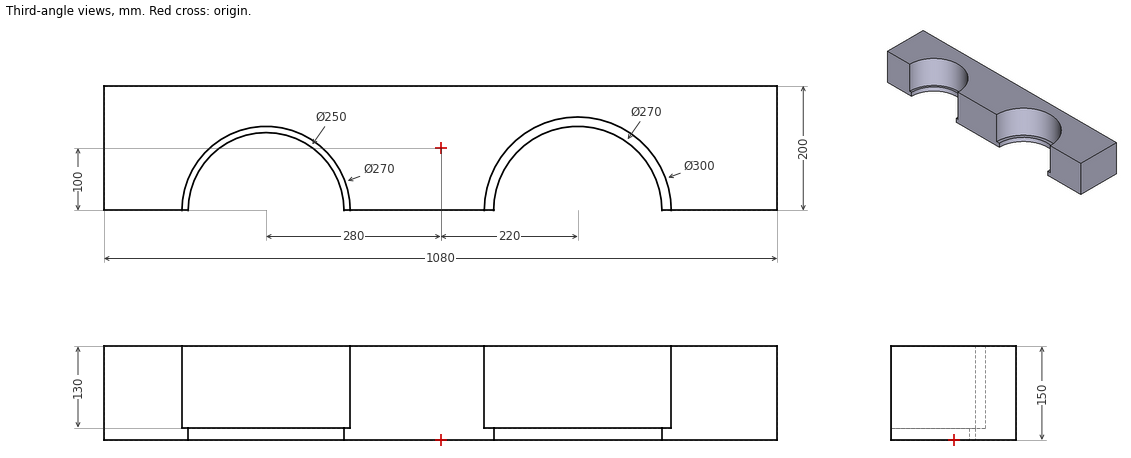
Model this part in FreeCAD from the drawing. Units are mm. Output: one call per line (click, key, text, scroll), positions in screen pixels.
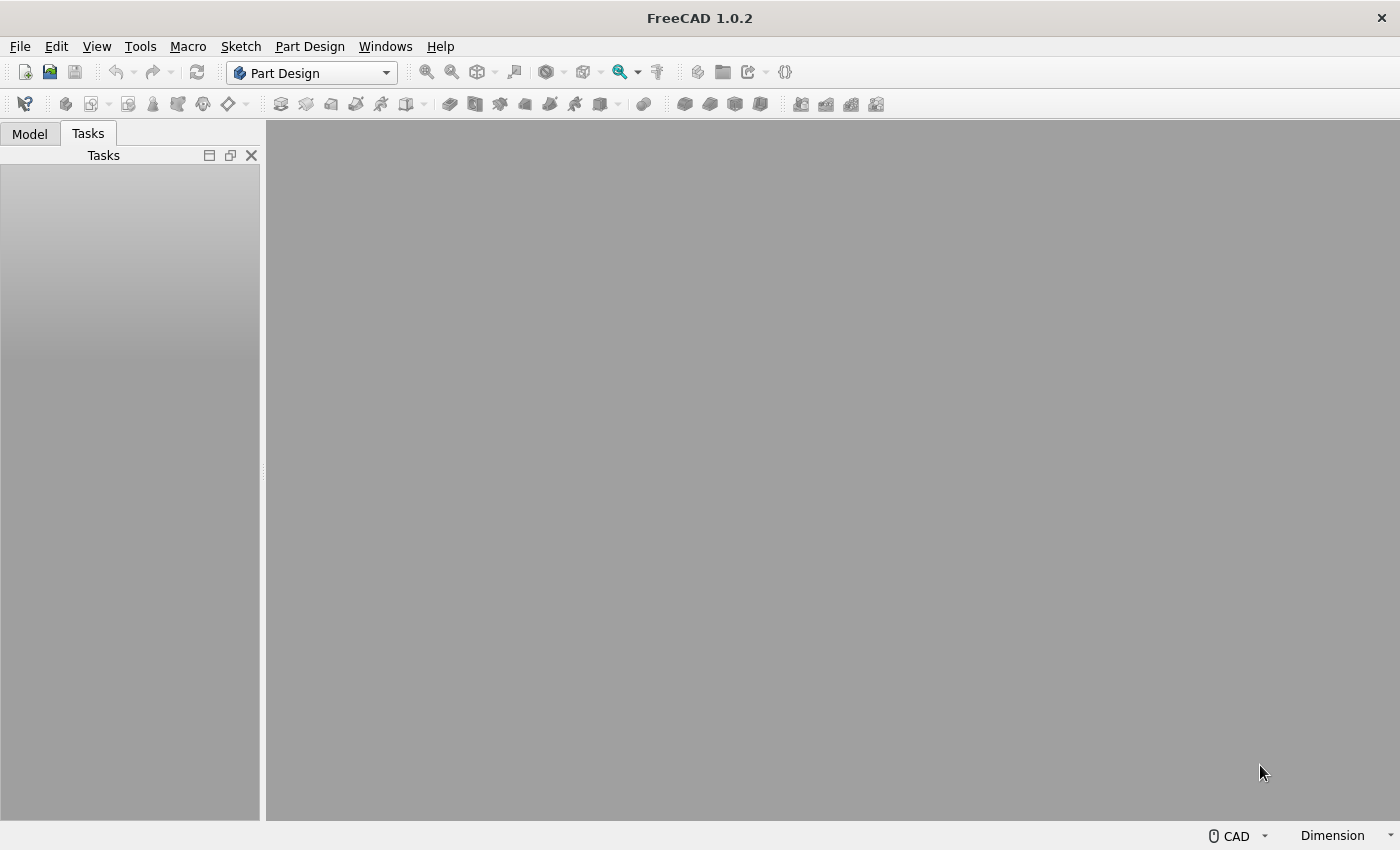
key(ctrl+n)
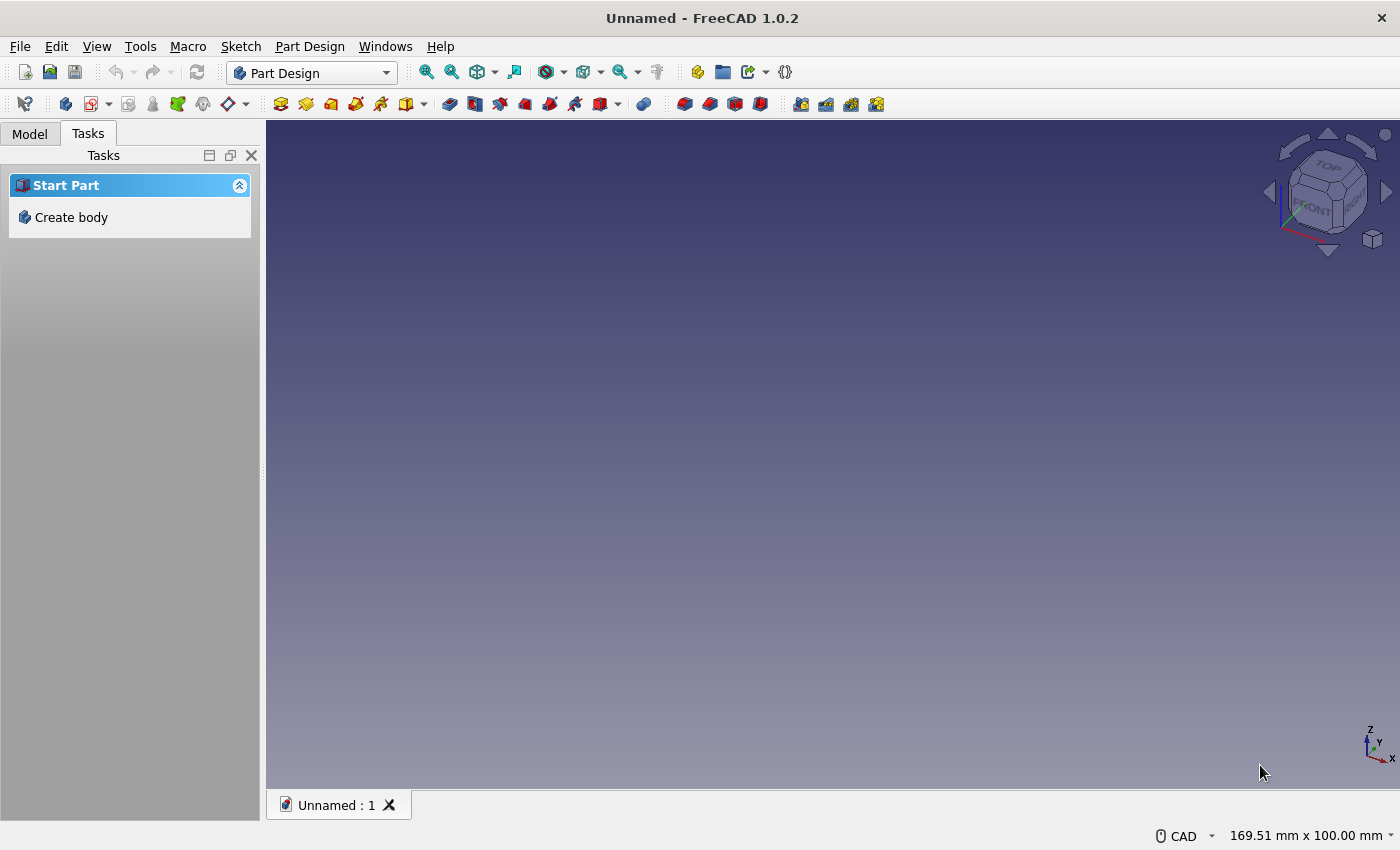
click(90, 104)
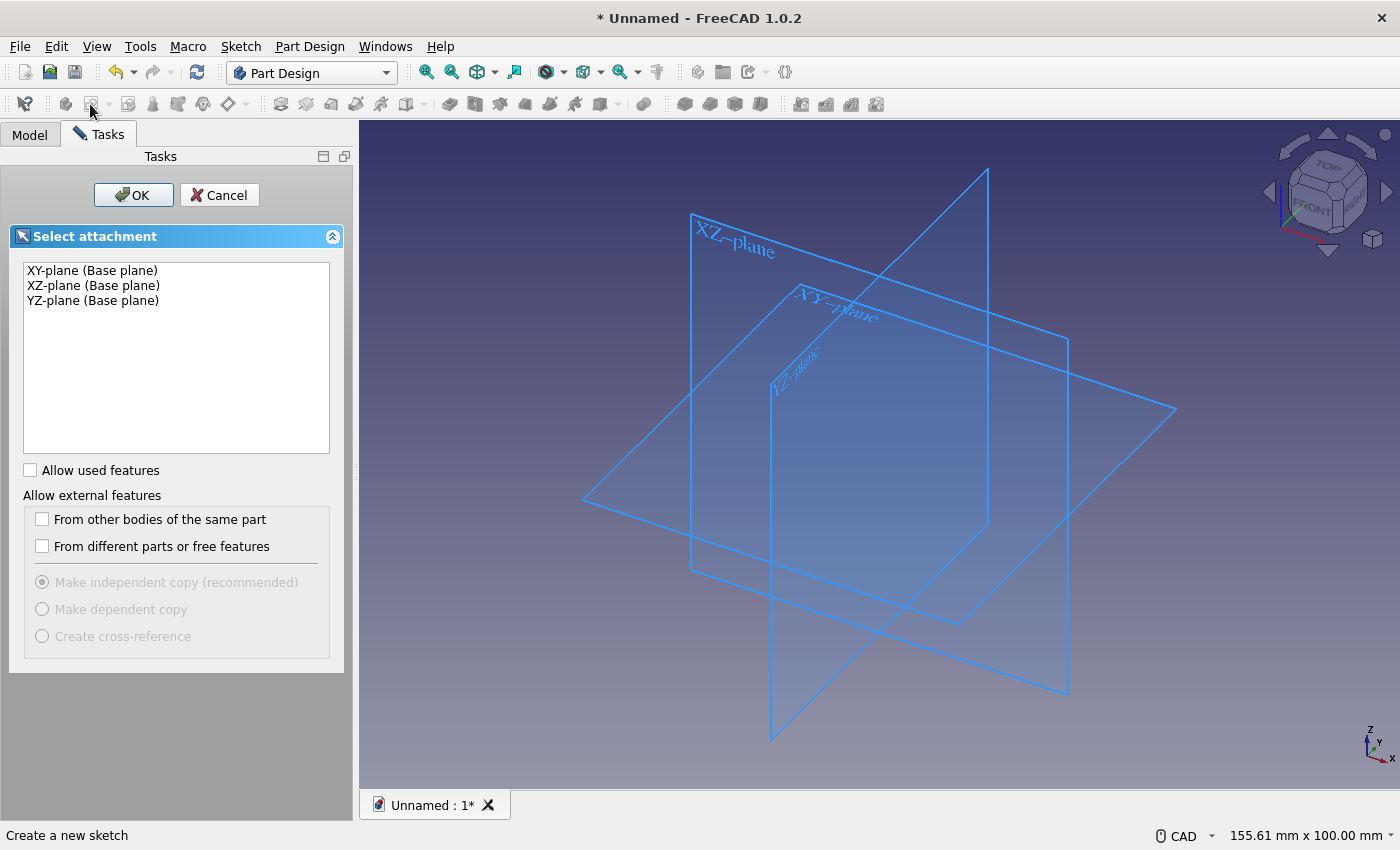
click(84, 270)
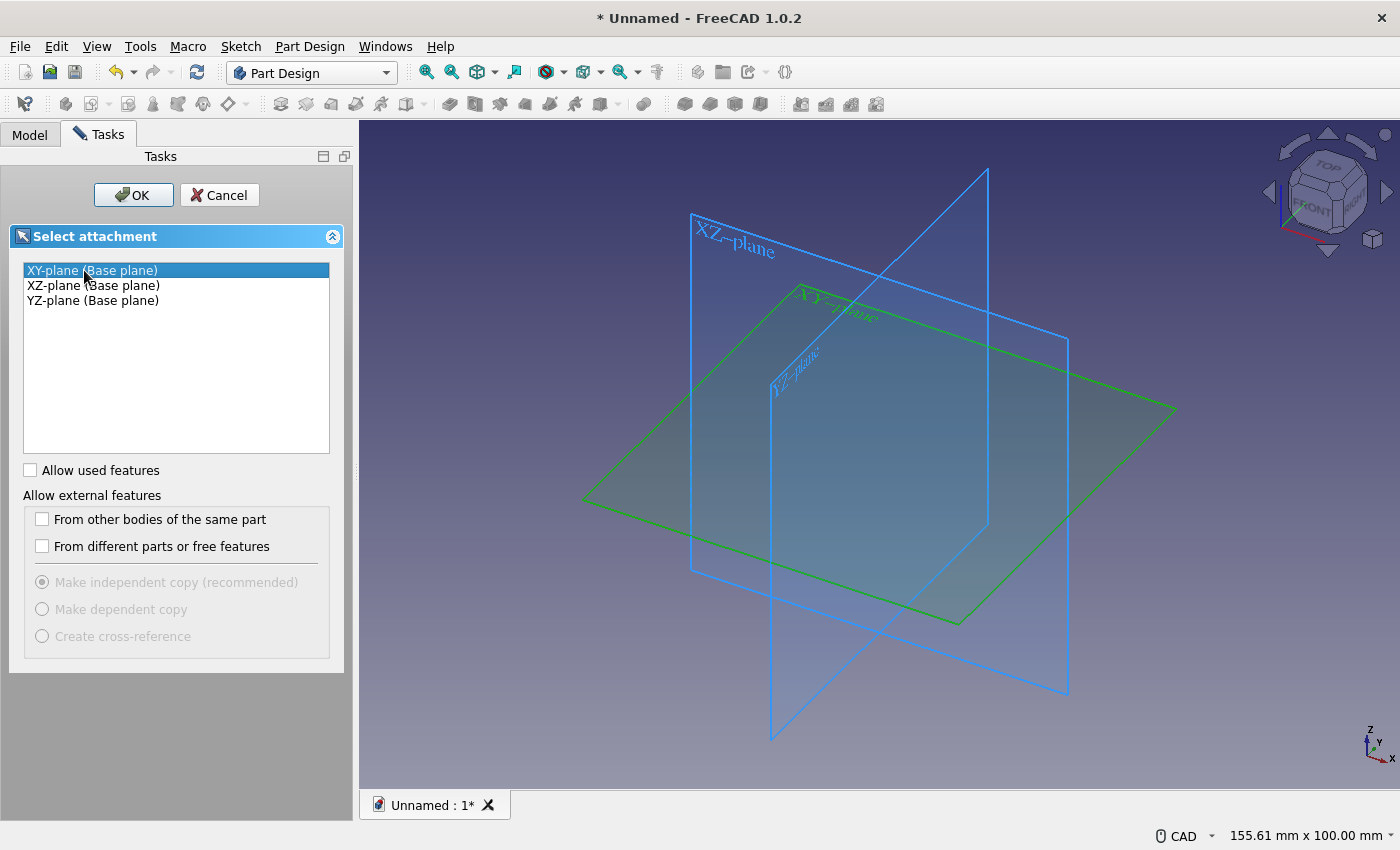
click(134, 195)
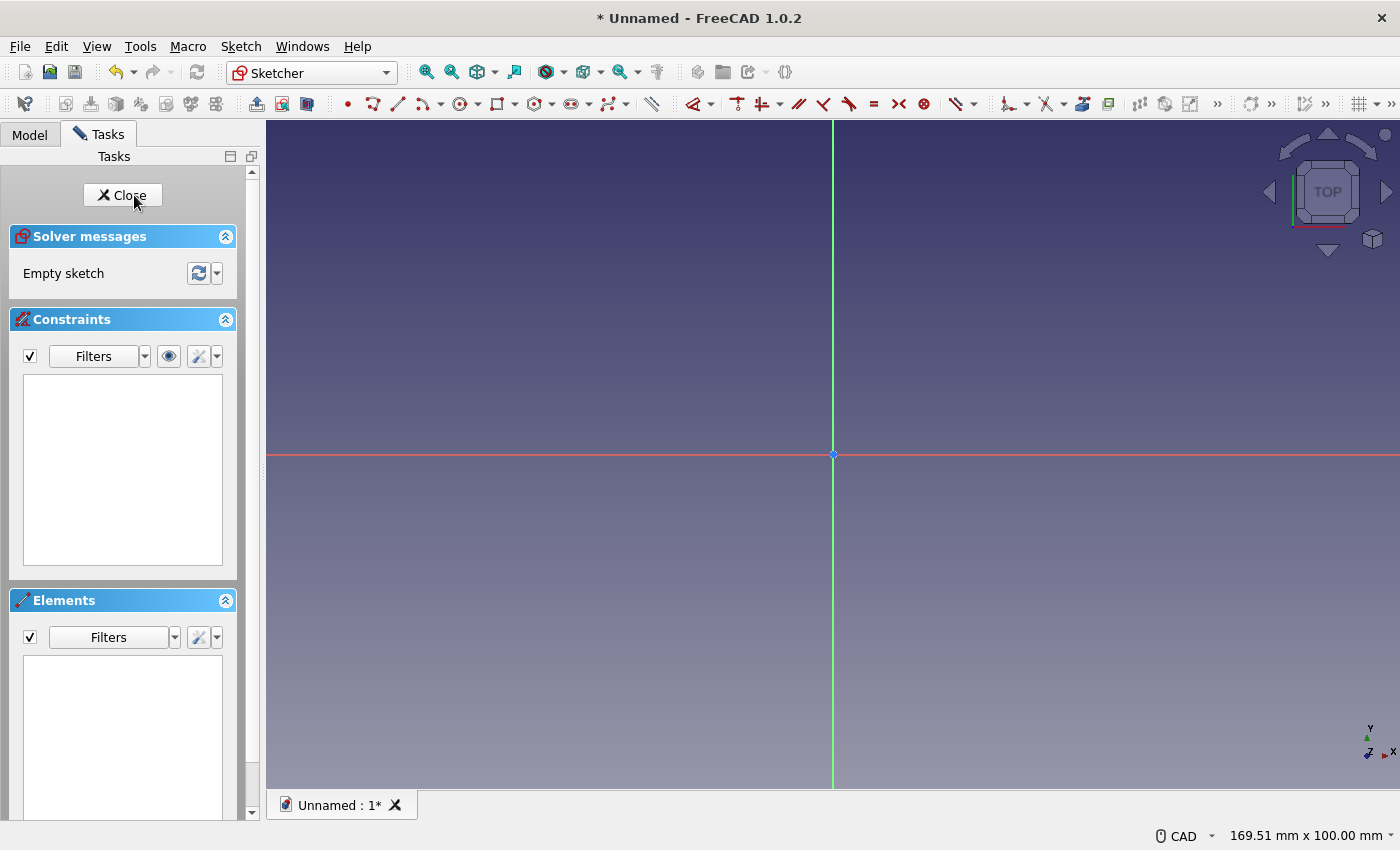
scroll(758, 454, down, 12)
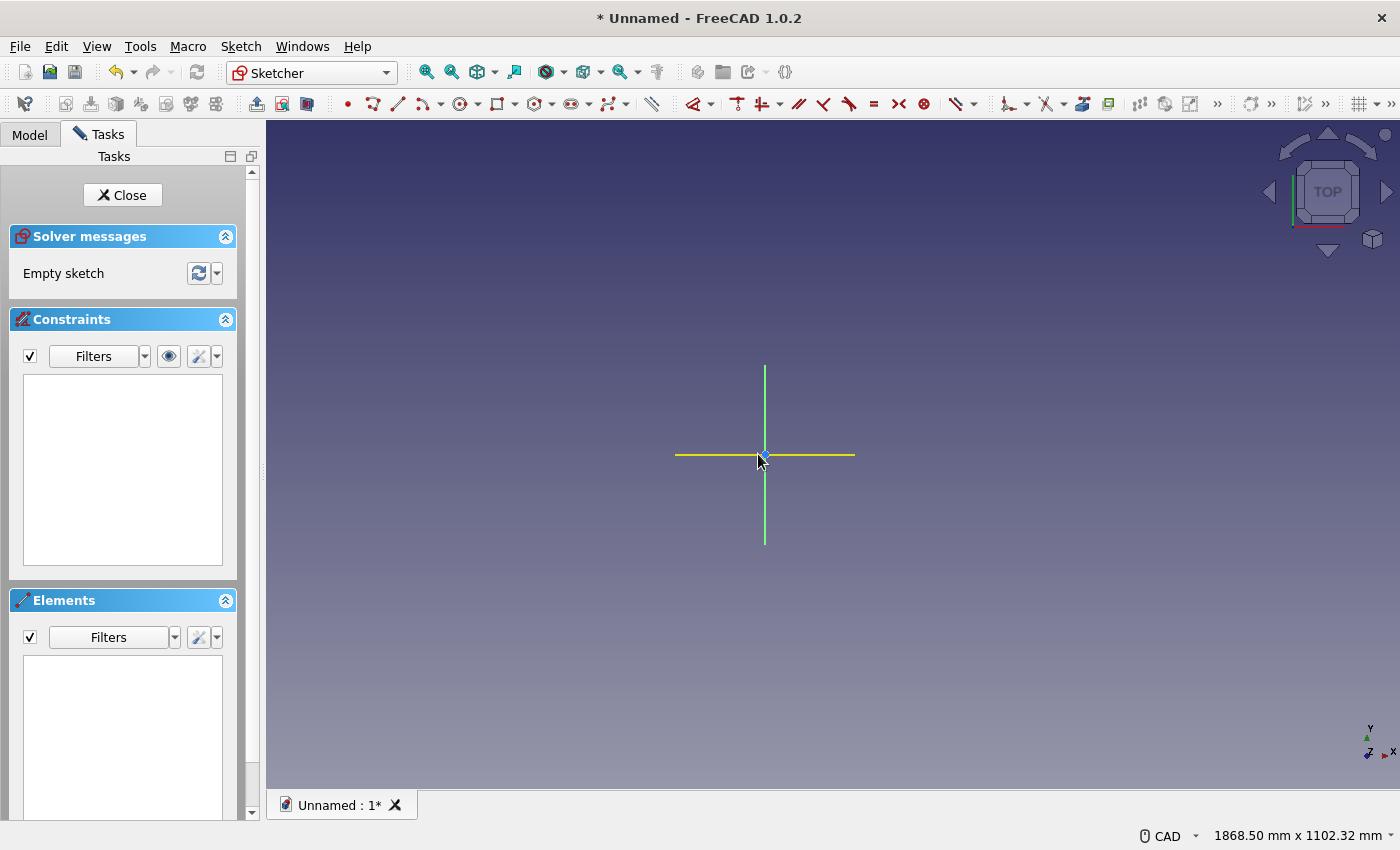
key(g)
key(v)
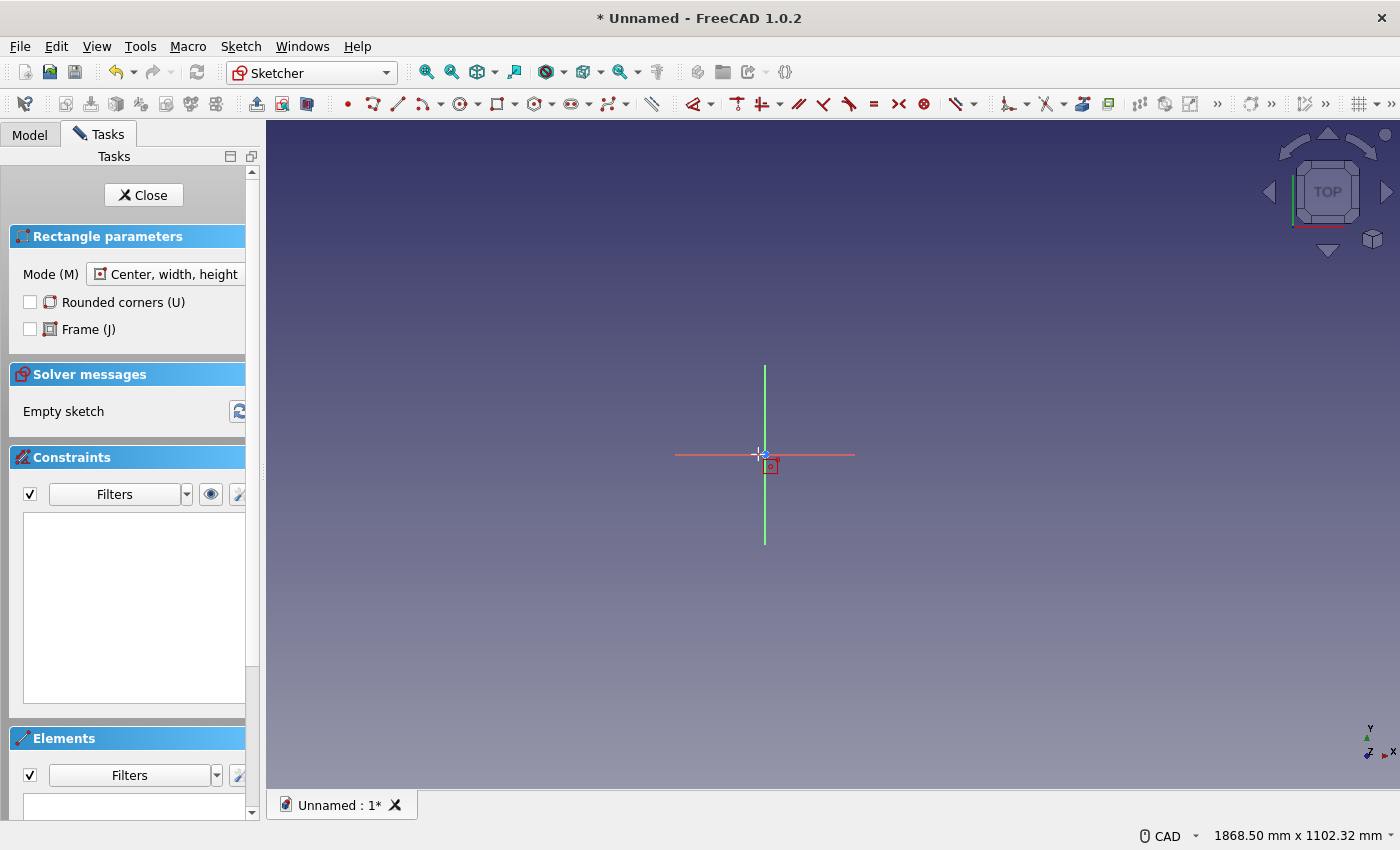
click(765, 454)
click(1093, 394)
key(Escape)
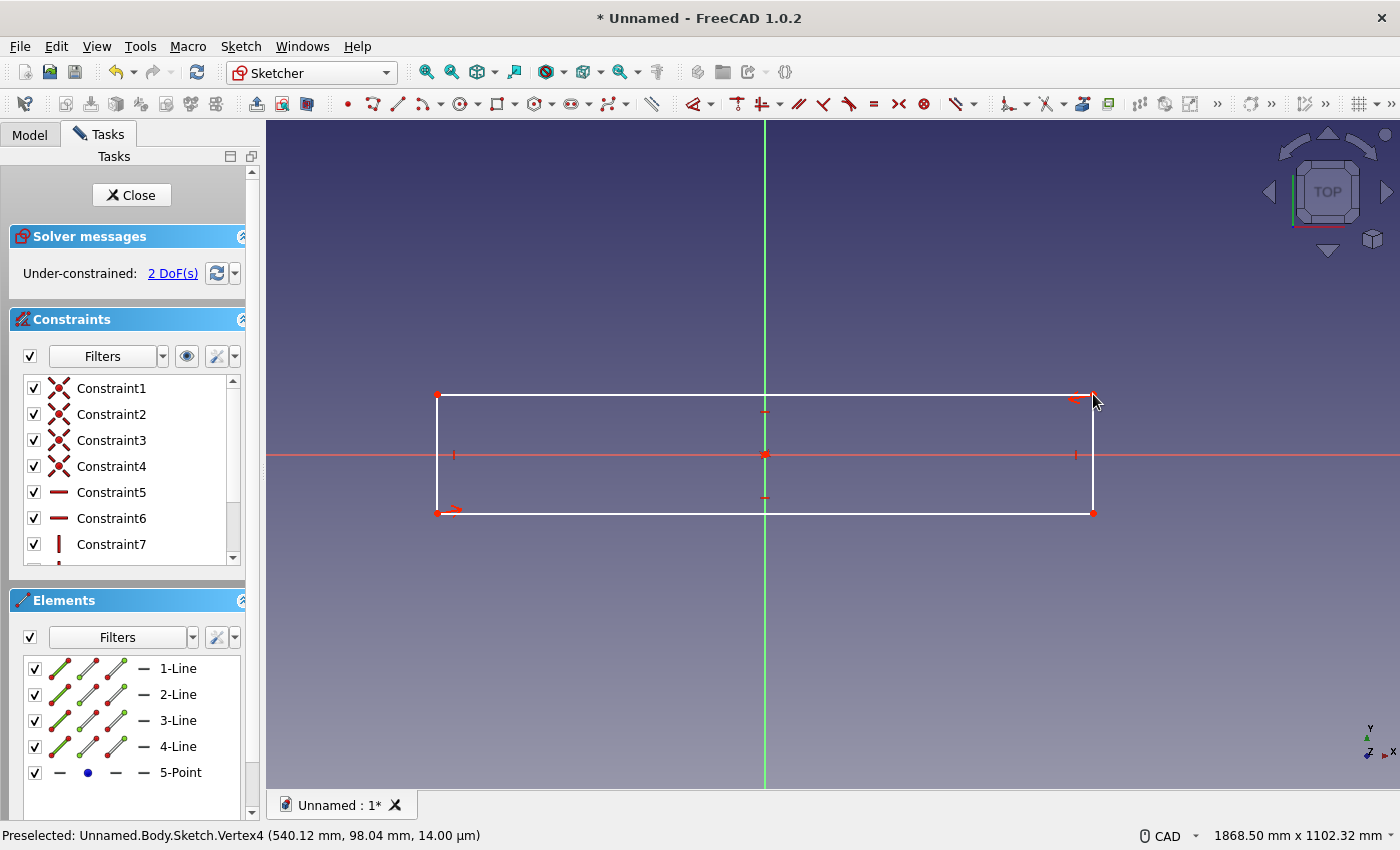
click(692, 104)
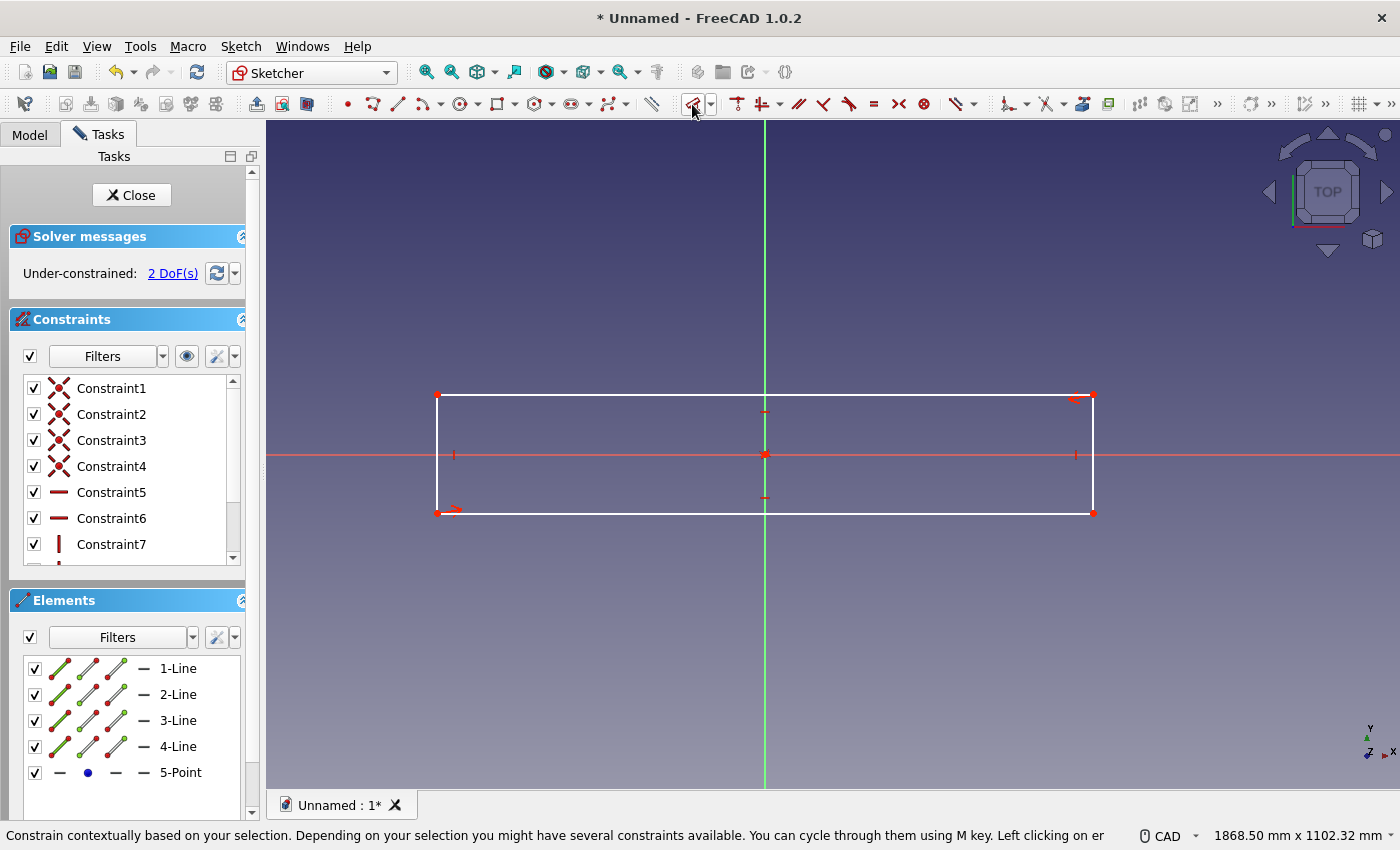
click(1093, 478)
click(1127, 427)